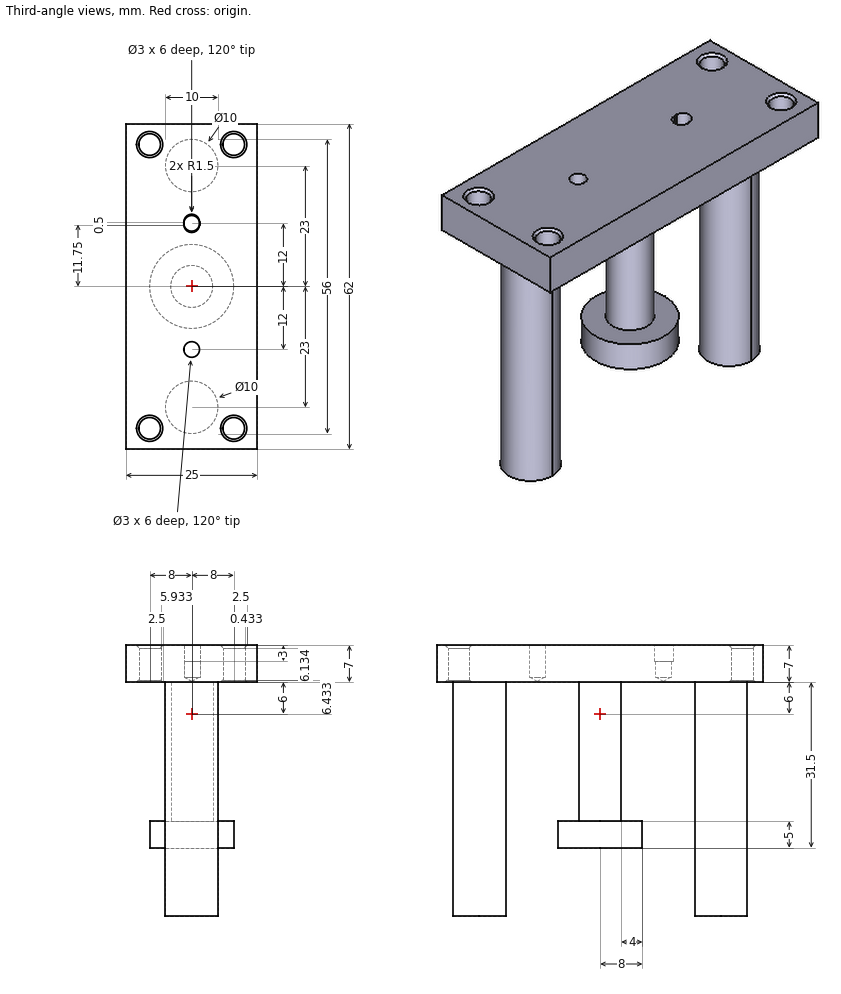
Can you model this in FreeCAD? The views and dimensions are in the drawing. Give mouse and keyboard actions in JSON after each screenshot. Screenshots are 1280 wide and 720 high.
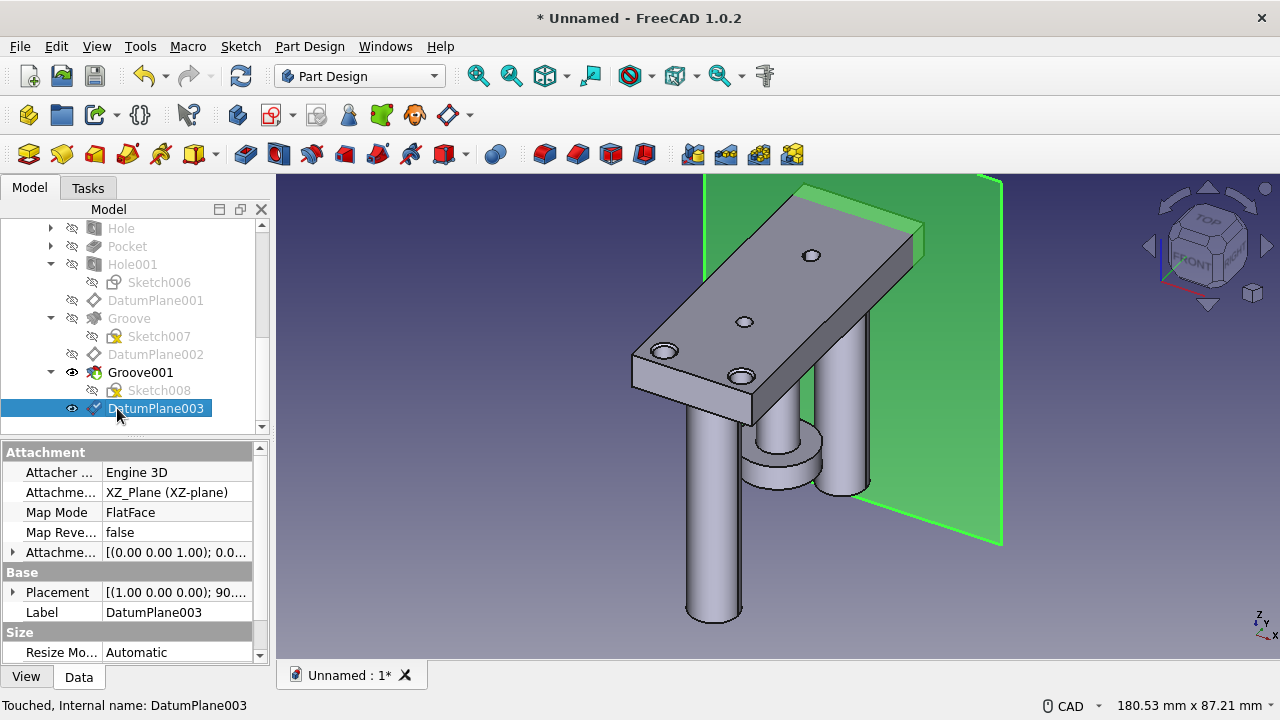
{"action": "left_click", "coordinate": [270, 116]}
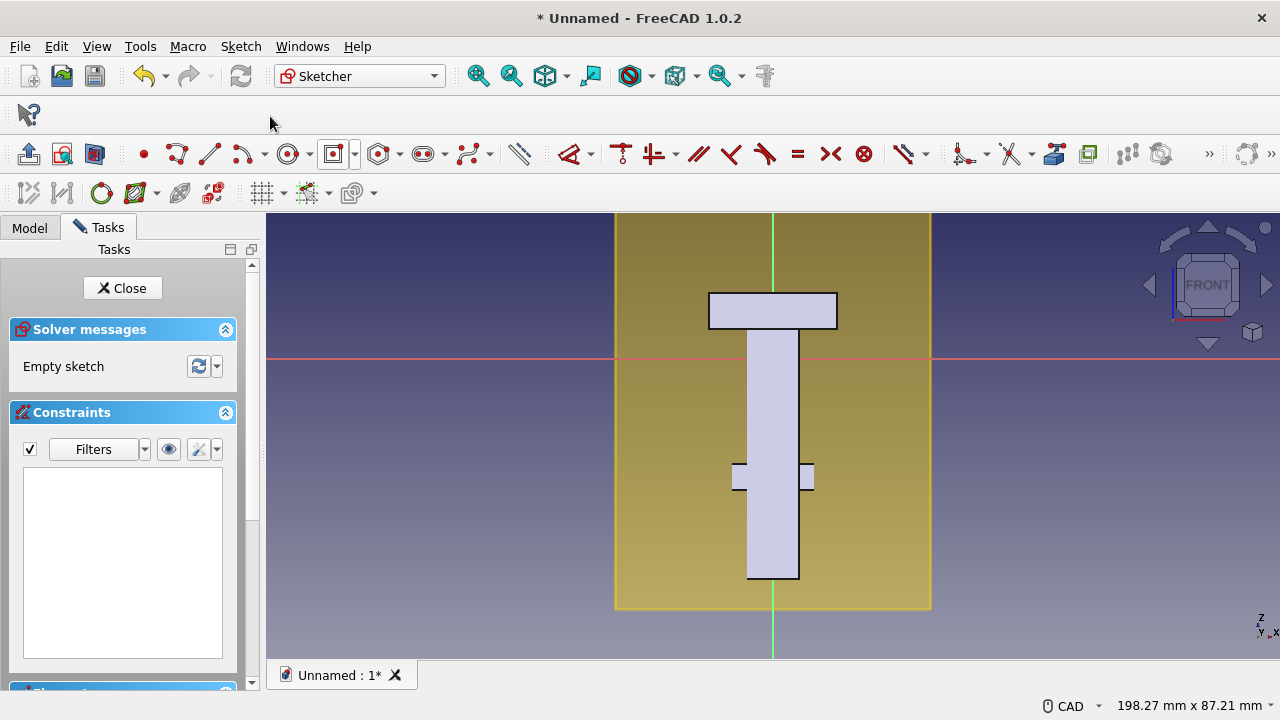
{"action": "left_click", "coordinate": [95, 154]}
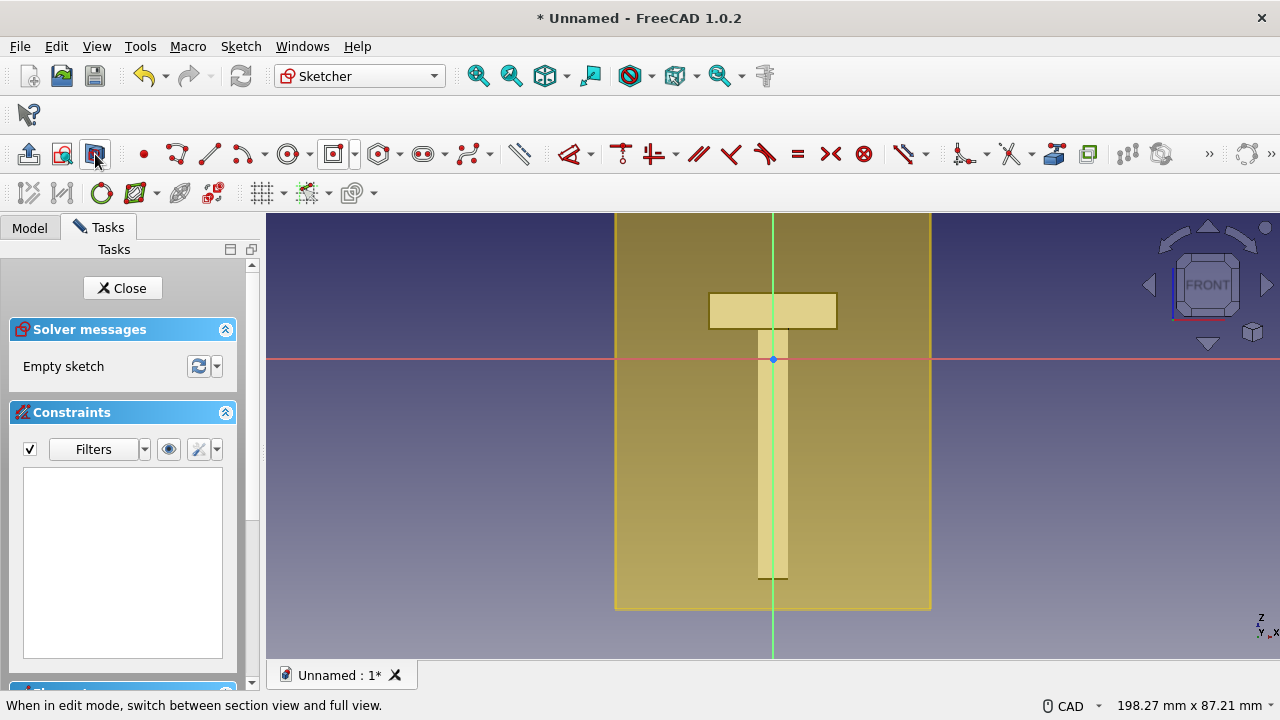
{"action": "scroll", "coordinate": [831, 290], "scroll_direction": "up", "scroll_amount": 7}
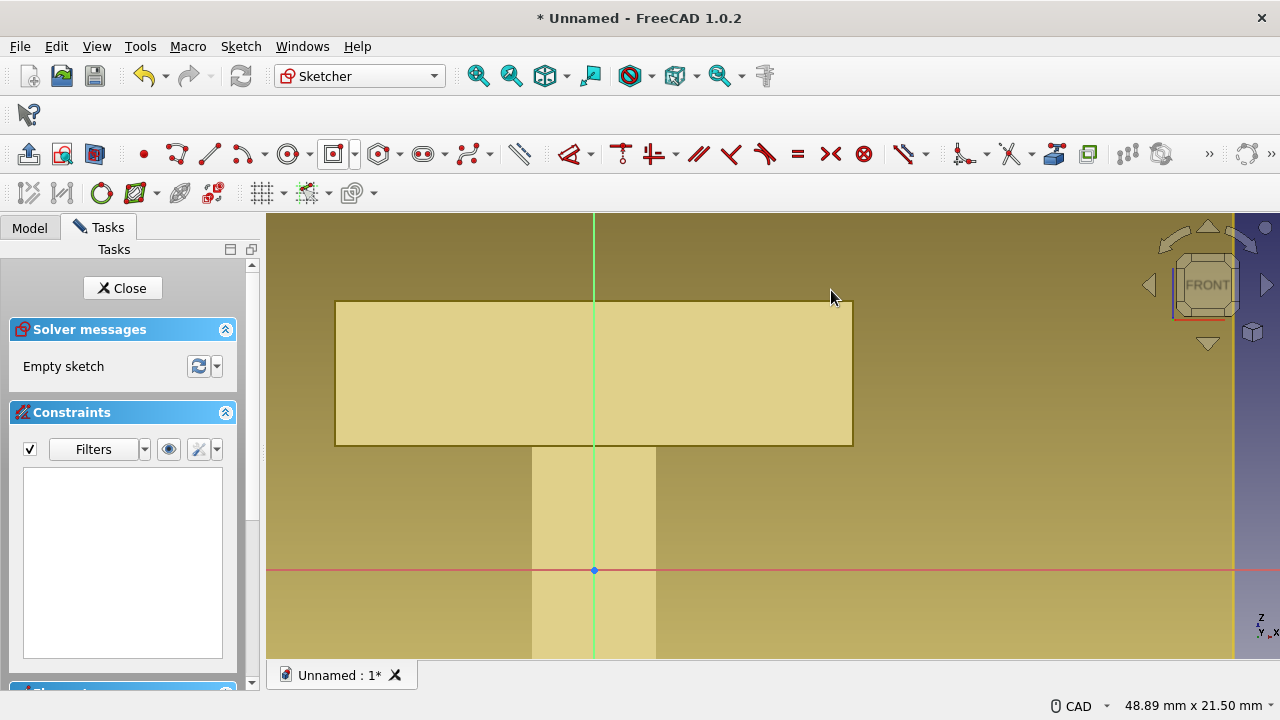
{"action": "left_click", "coordinate": [177, 154]}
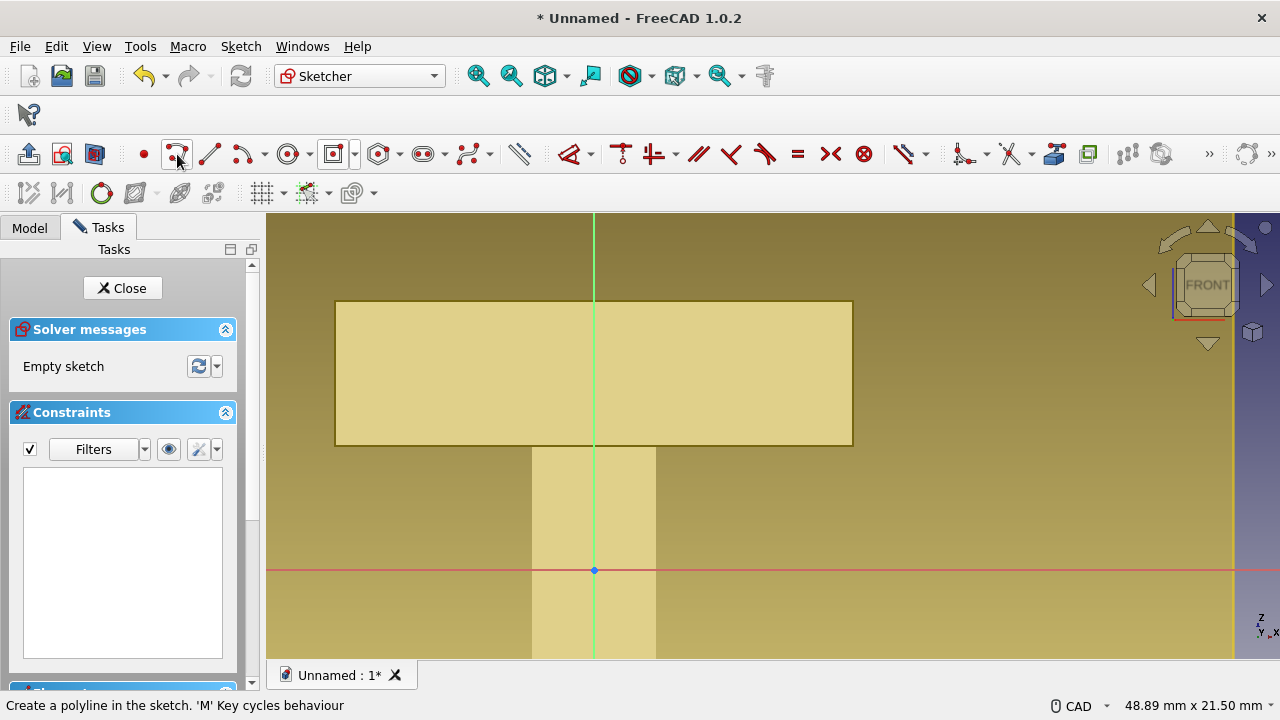
{"action": "left_click", "coordinate": [760, 446]}
{"action": "left_click", "coordinate": [760, 301]}
{"action": "left_click", "coordinate": [812, 301]}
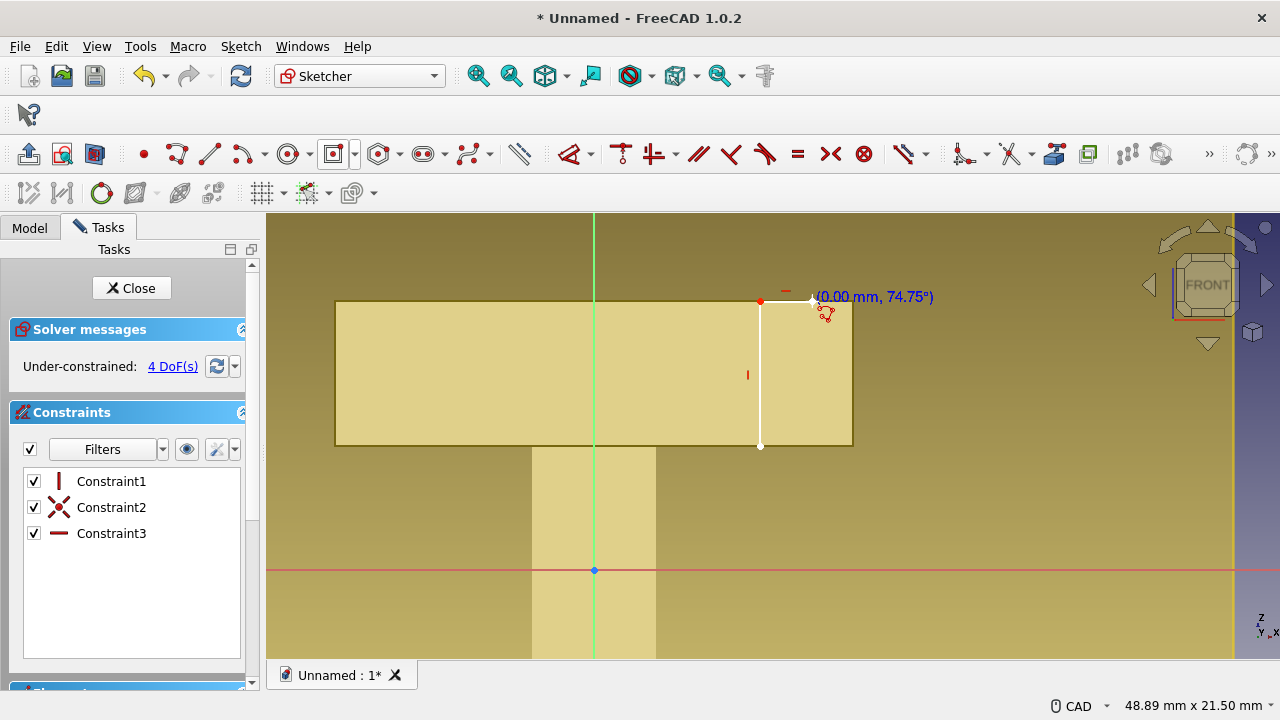
{"action": "scroll", "coordinate": [803, 310], "scroll_direction": "up", "scroll_amount": 3}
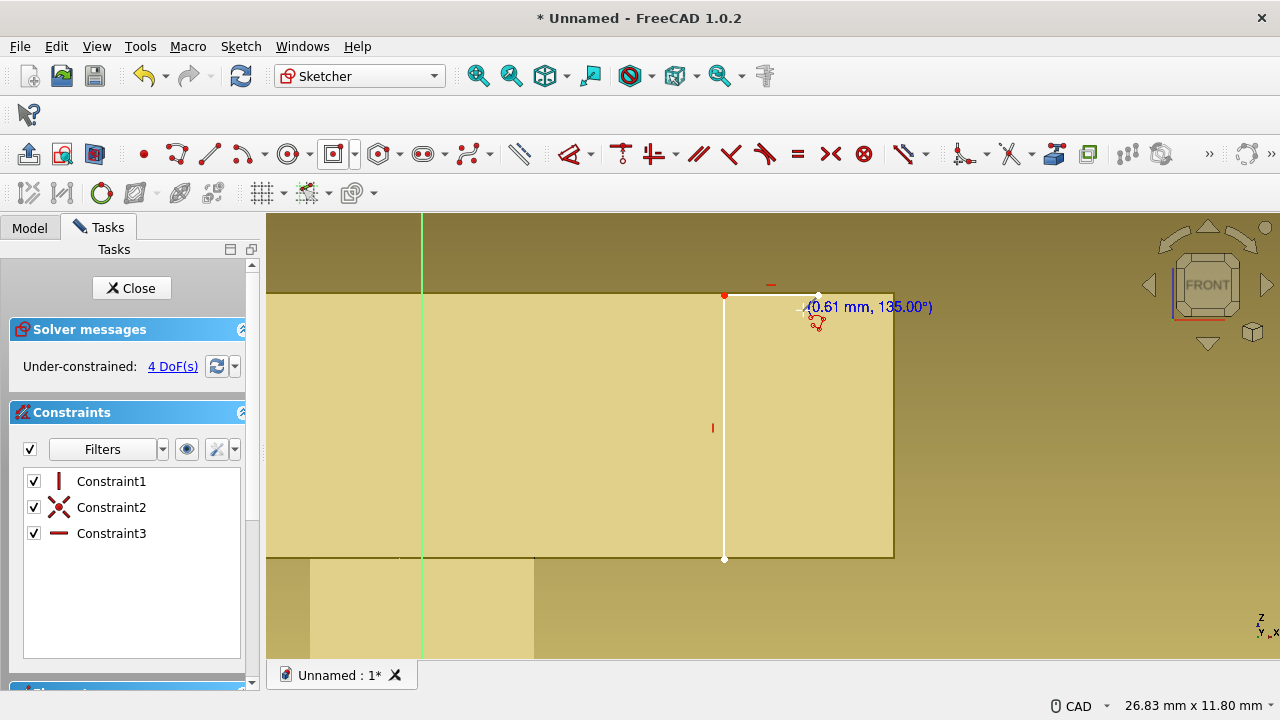
{"action": "left_click", "coordinate": [802, 309]}
{"action": "left_click", "coordinate": [802, 541]}
{"action": "left_click", "coordinate": [819, 558]}
{"action": "left_click", "coordinate": [724, 559]}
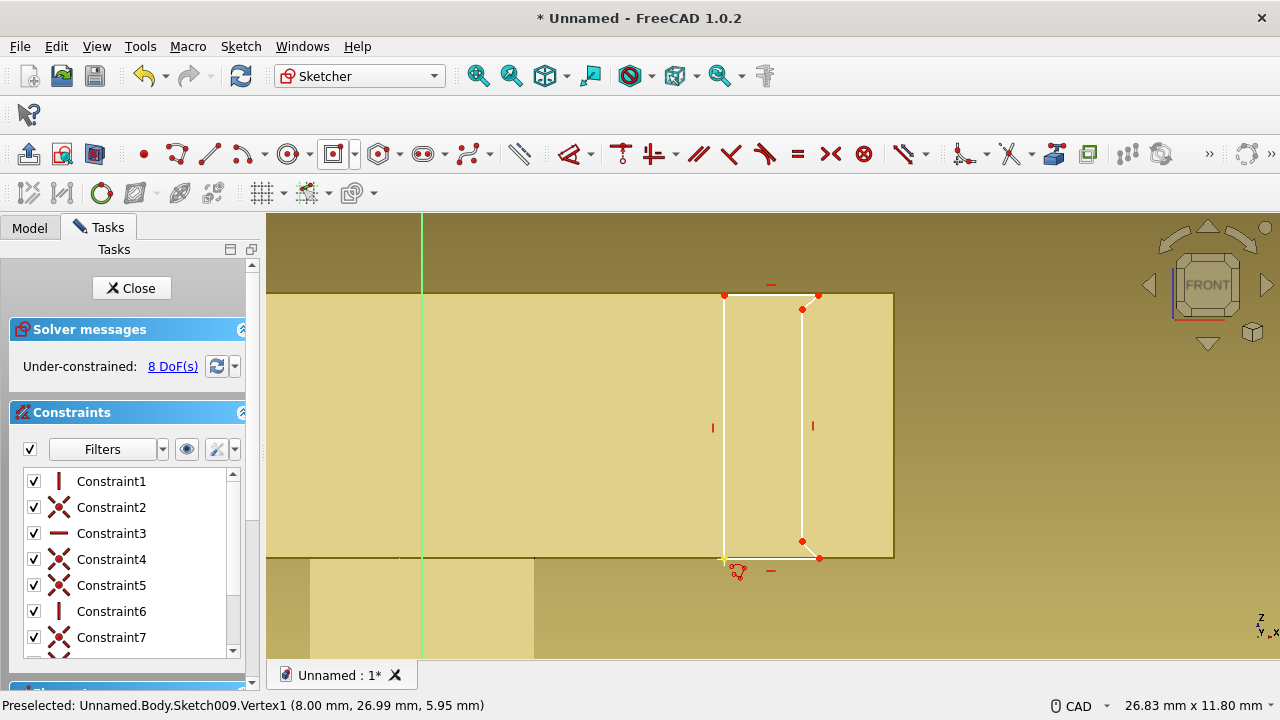
{"action": "left_click", "coordinate": [210, 154]}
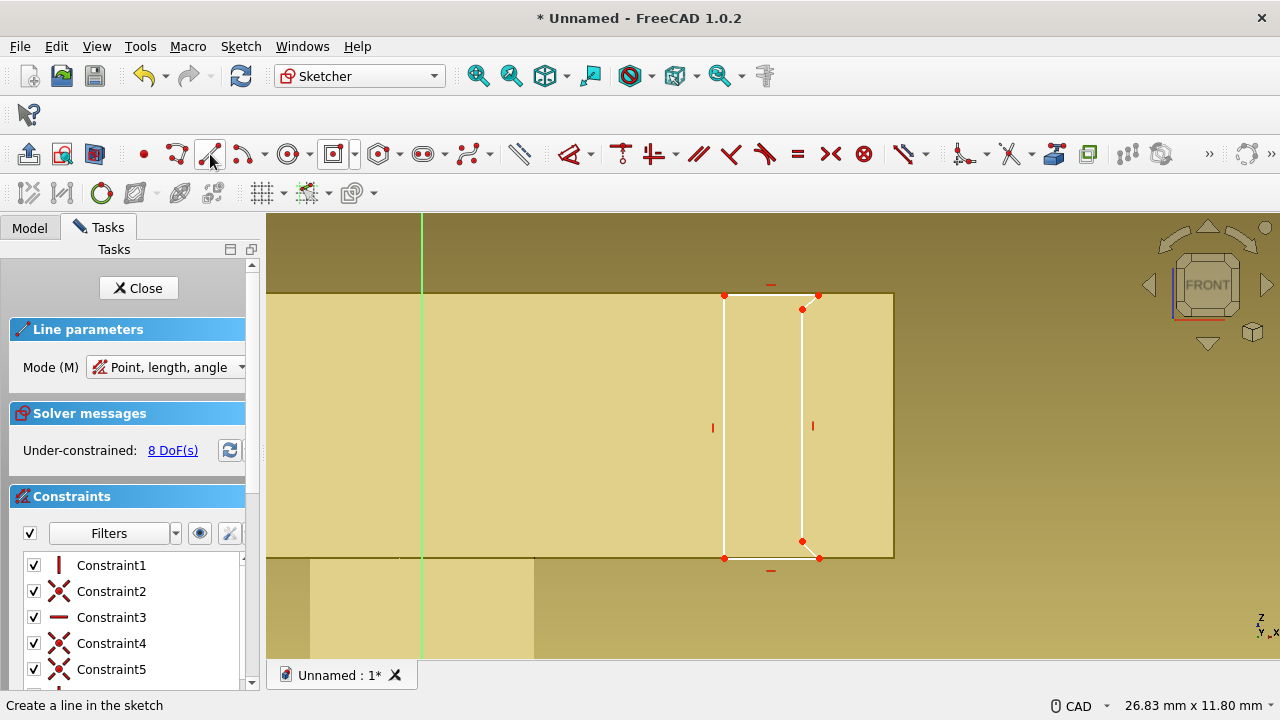
{"action": "left_click", "coordinate": [724, 584]}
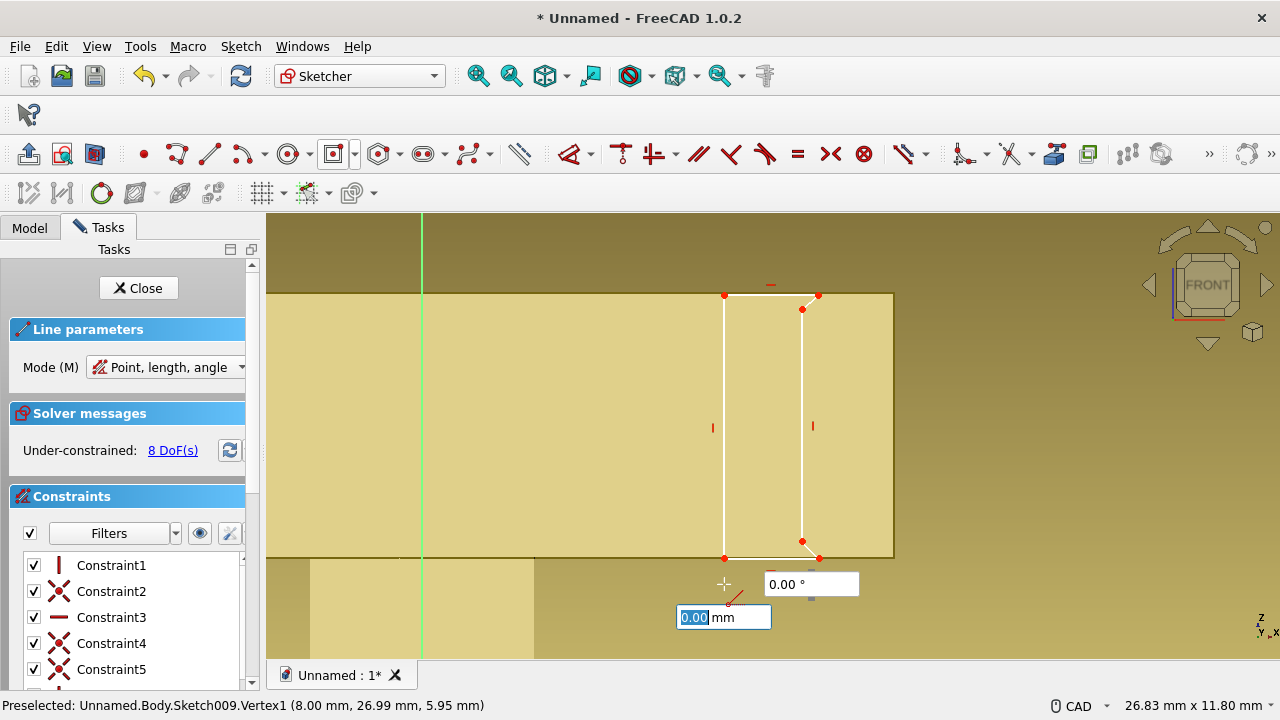
{"action": "scroll", "coordinate": [807, 311], "scroll_direction": "down", "scroll_amount": 3}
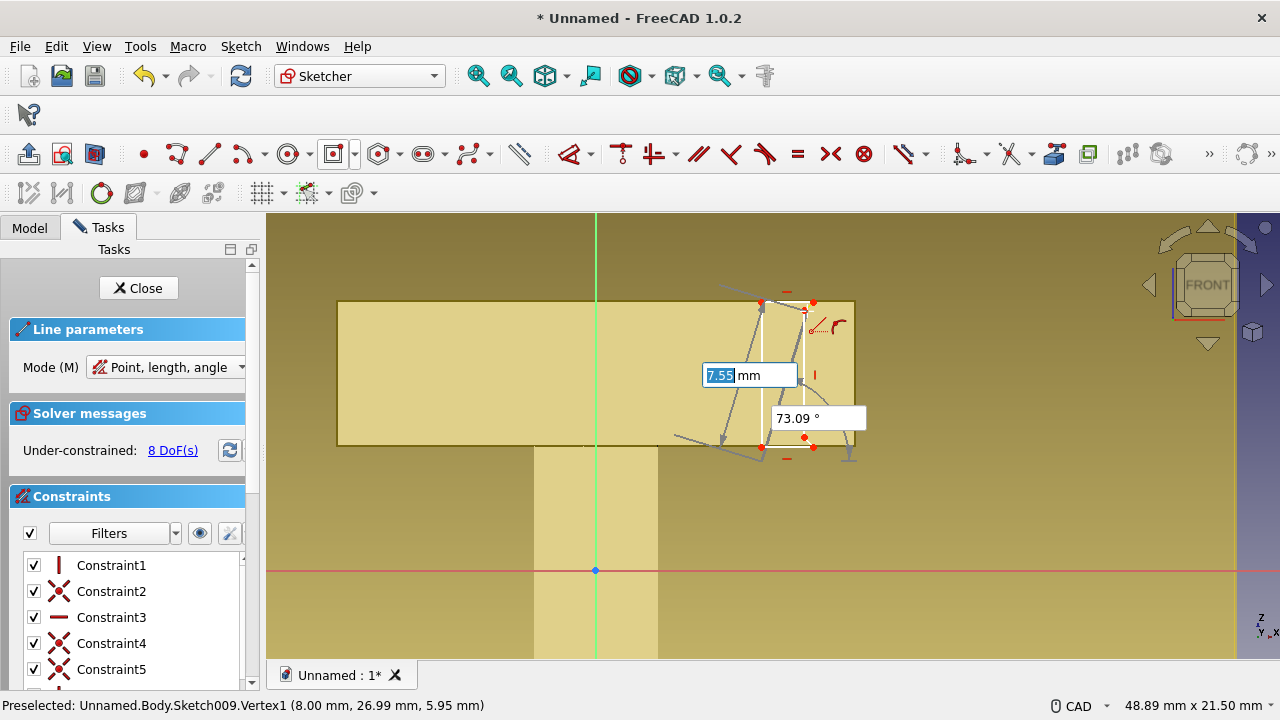
{"action": "left_click", "coordinate": [762, 505]}
{"action": "key", "text": "Escape"}